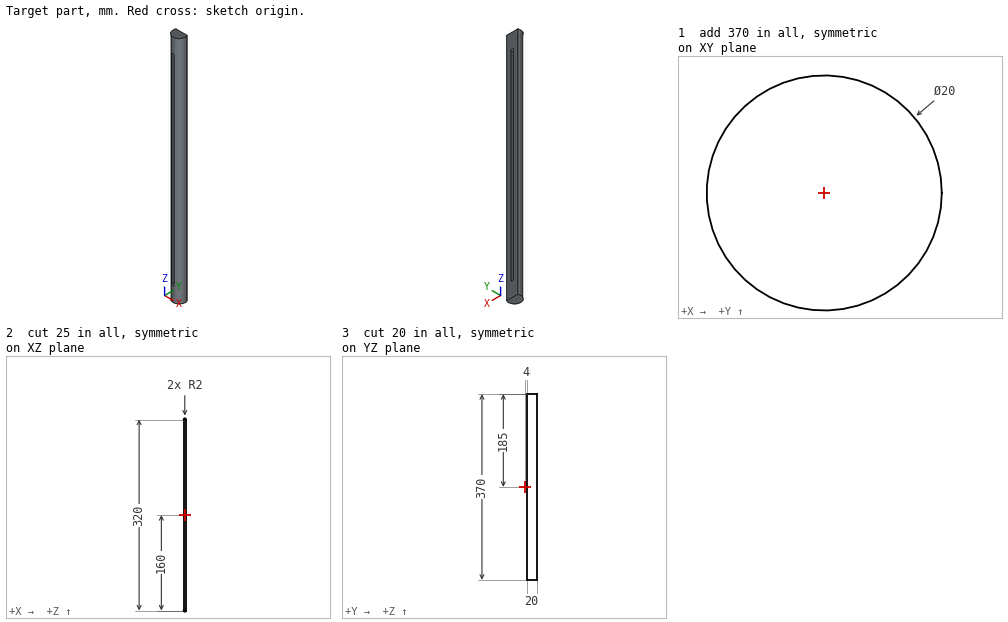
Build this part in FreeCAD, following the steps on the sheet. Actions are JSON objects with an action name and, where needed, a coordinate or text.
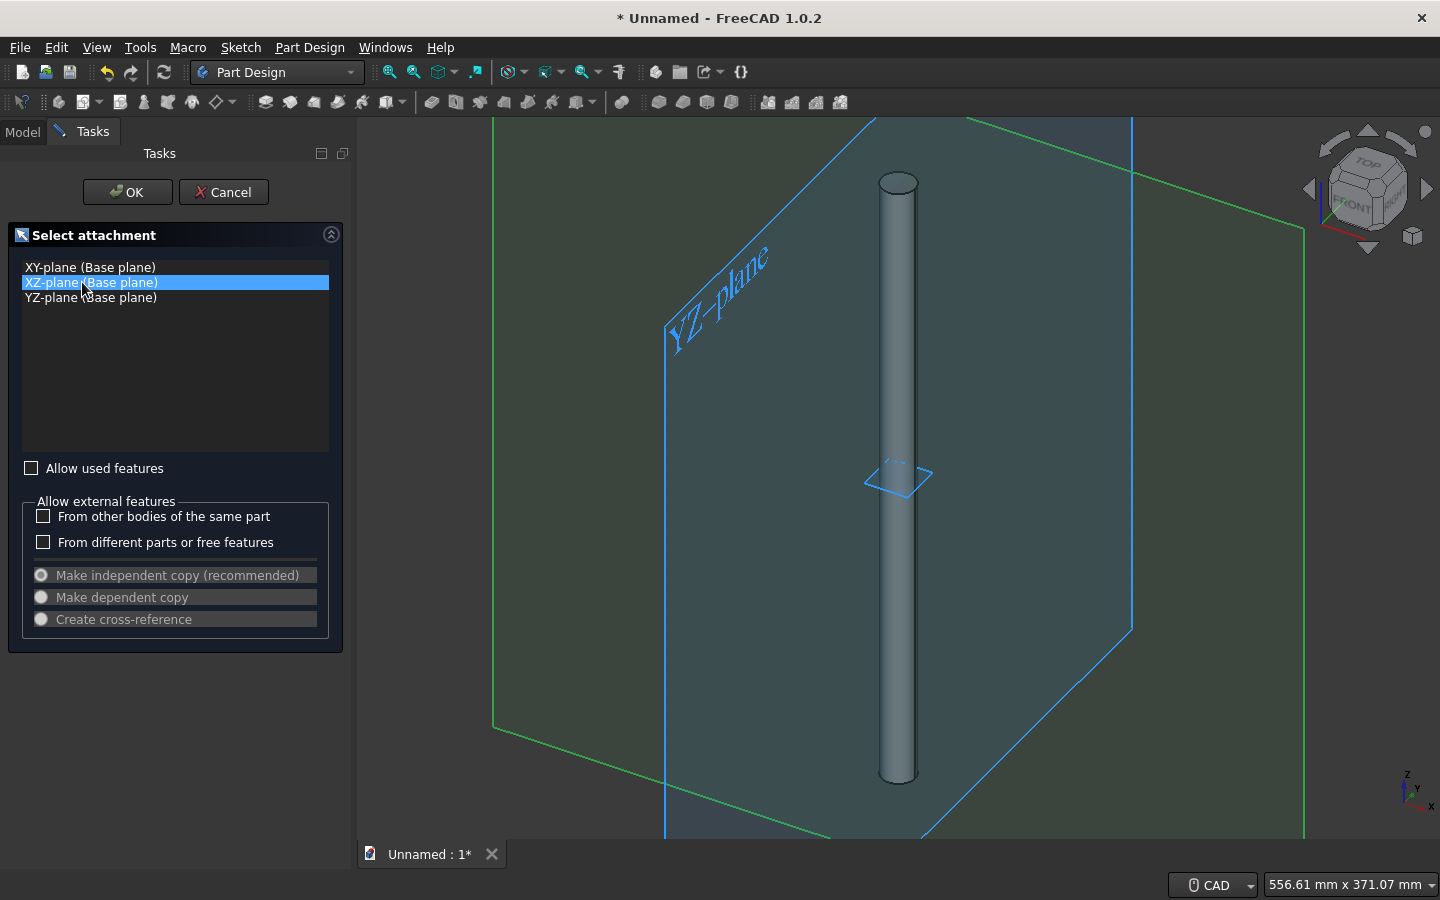
{"action": "left_click", "coordinate": [128, 192]}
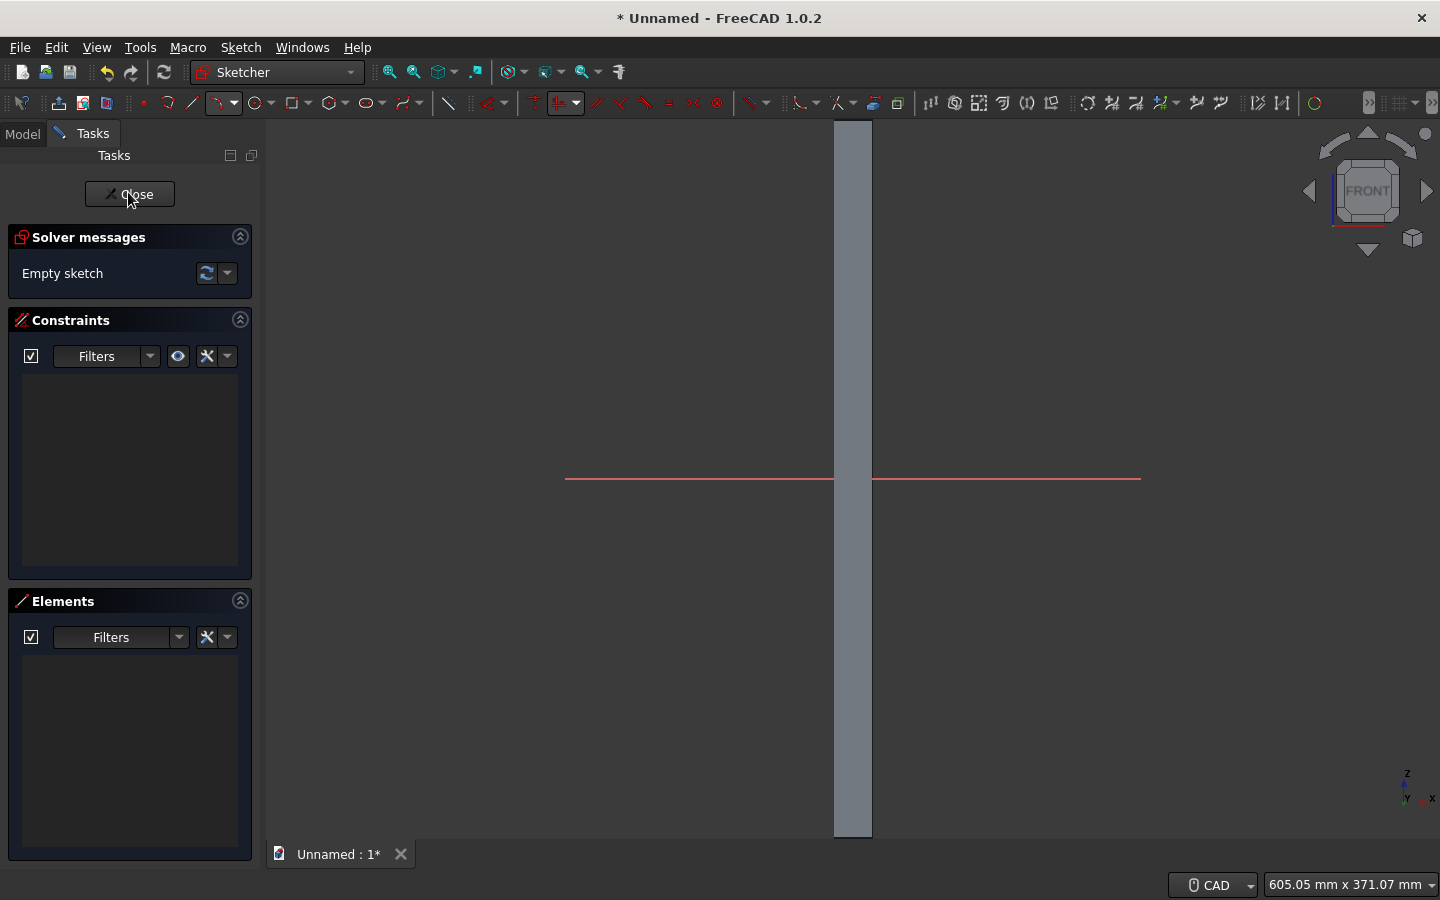
{"action": "left_click", "coordinate": [108, 104]}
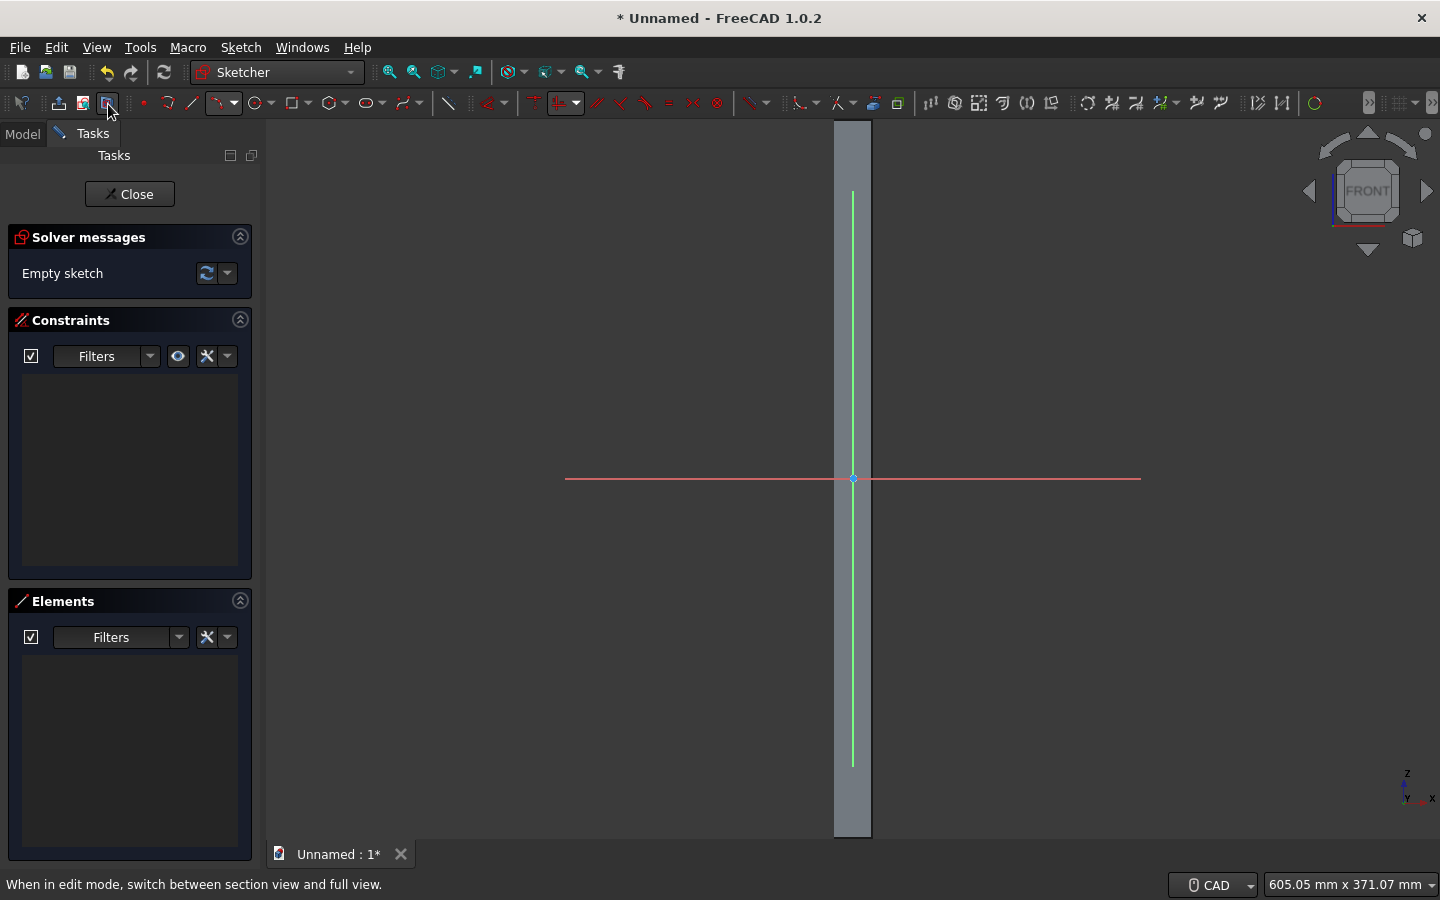
{"action": "scroll", "coordinate": [475, 479], "scroll_direction": "down", "scroll_amount": 1}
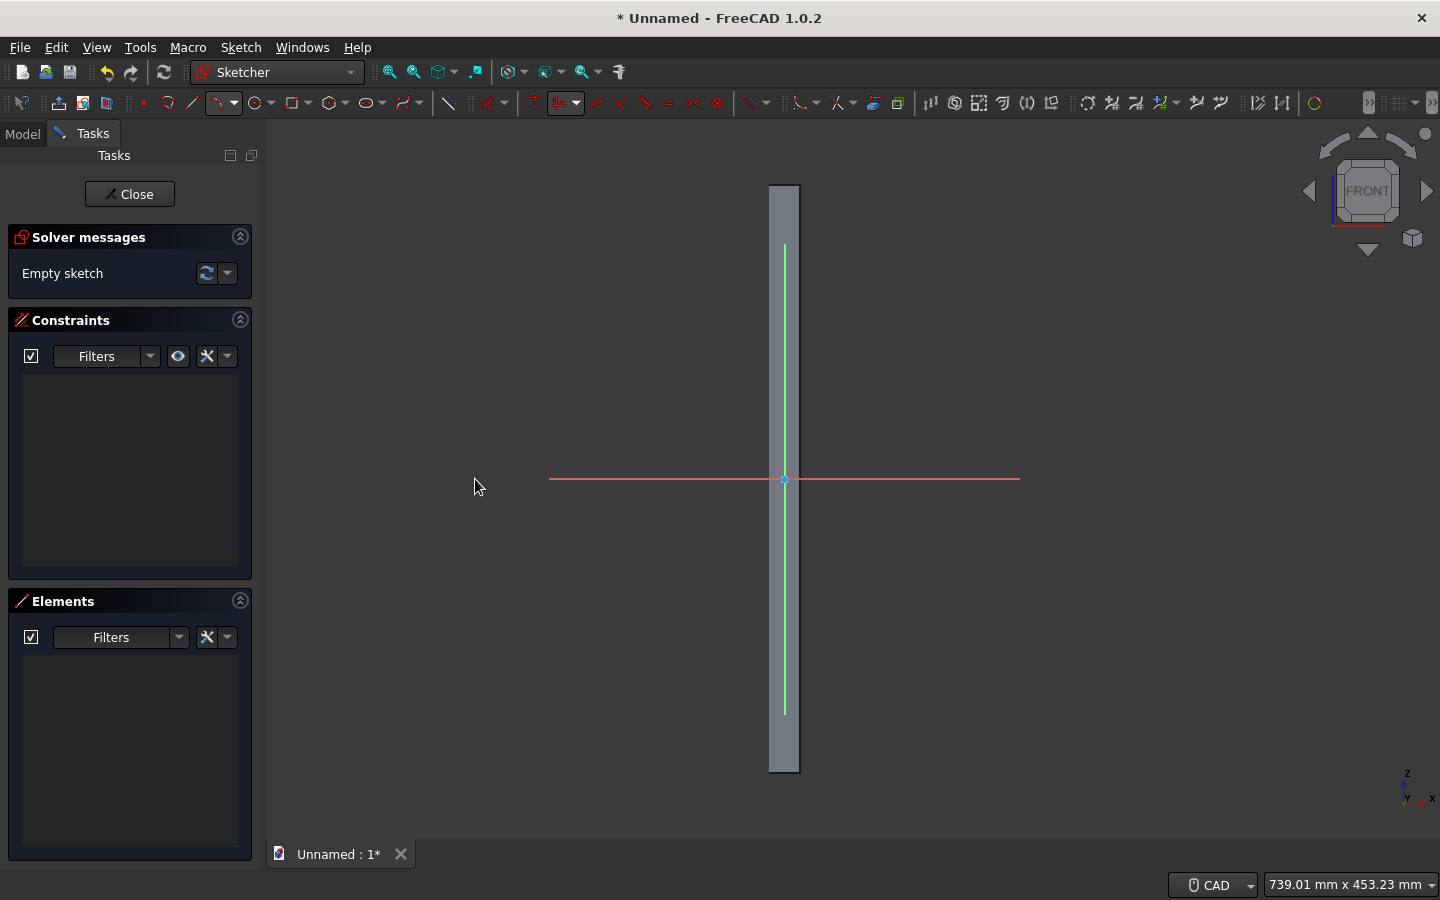
{"action": "left_click", "coordinate": [366, 104]}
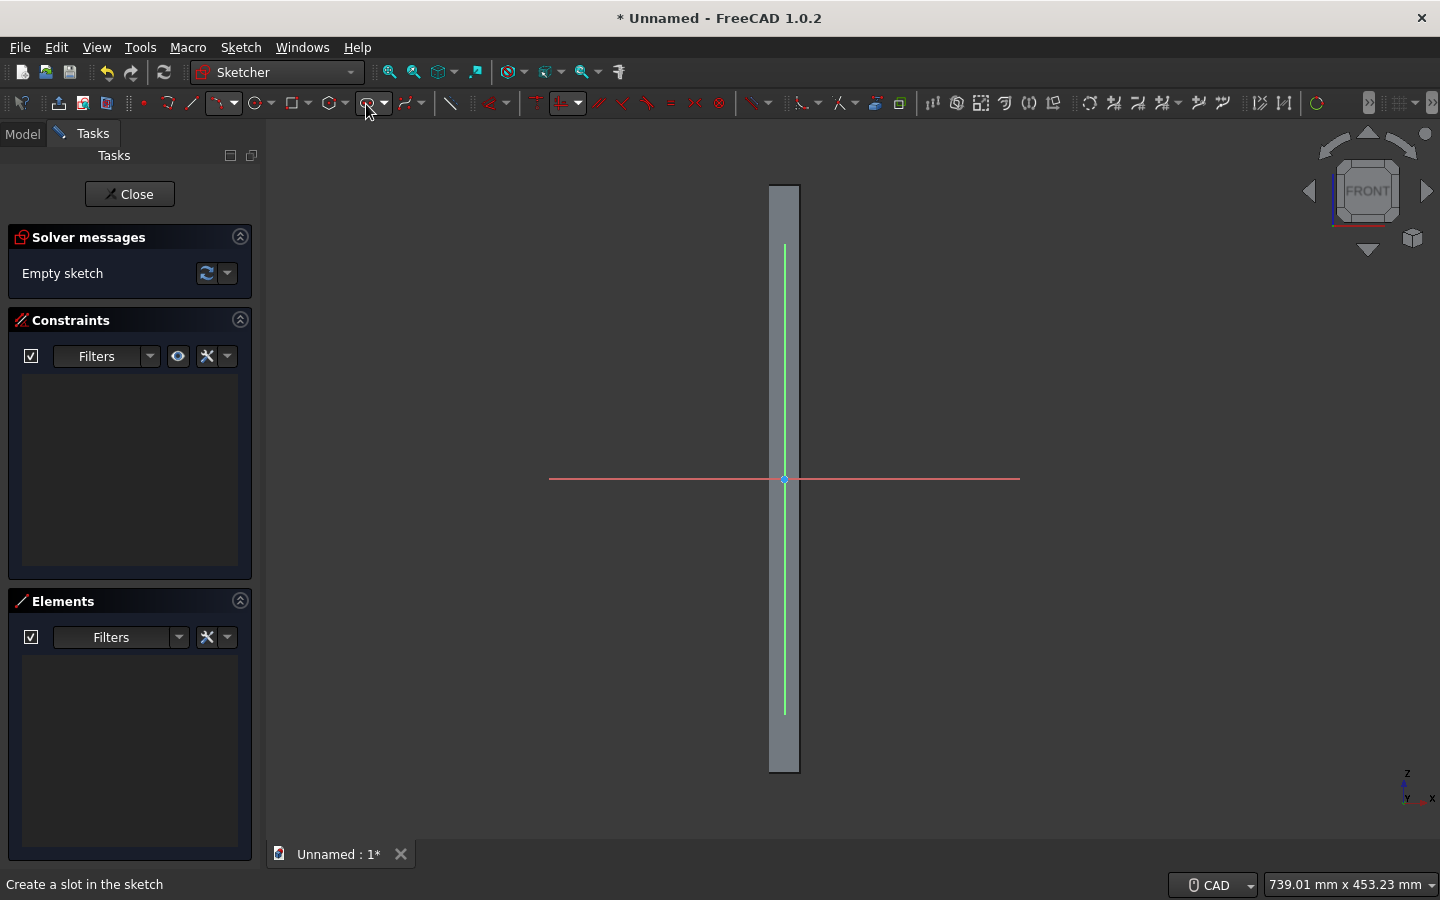
{"action": "scroll", "coordinate": [785, 733], "scroll_direction": "up", "scroll_amount": 10}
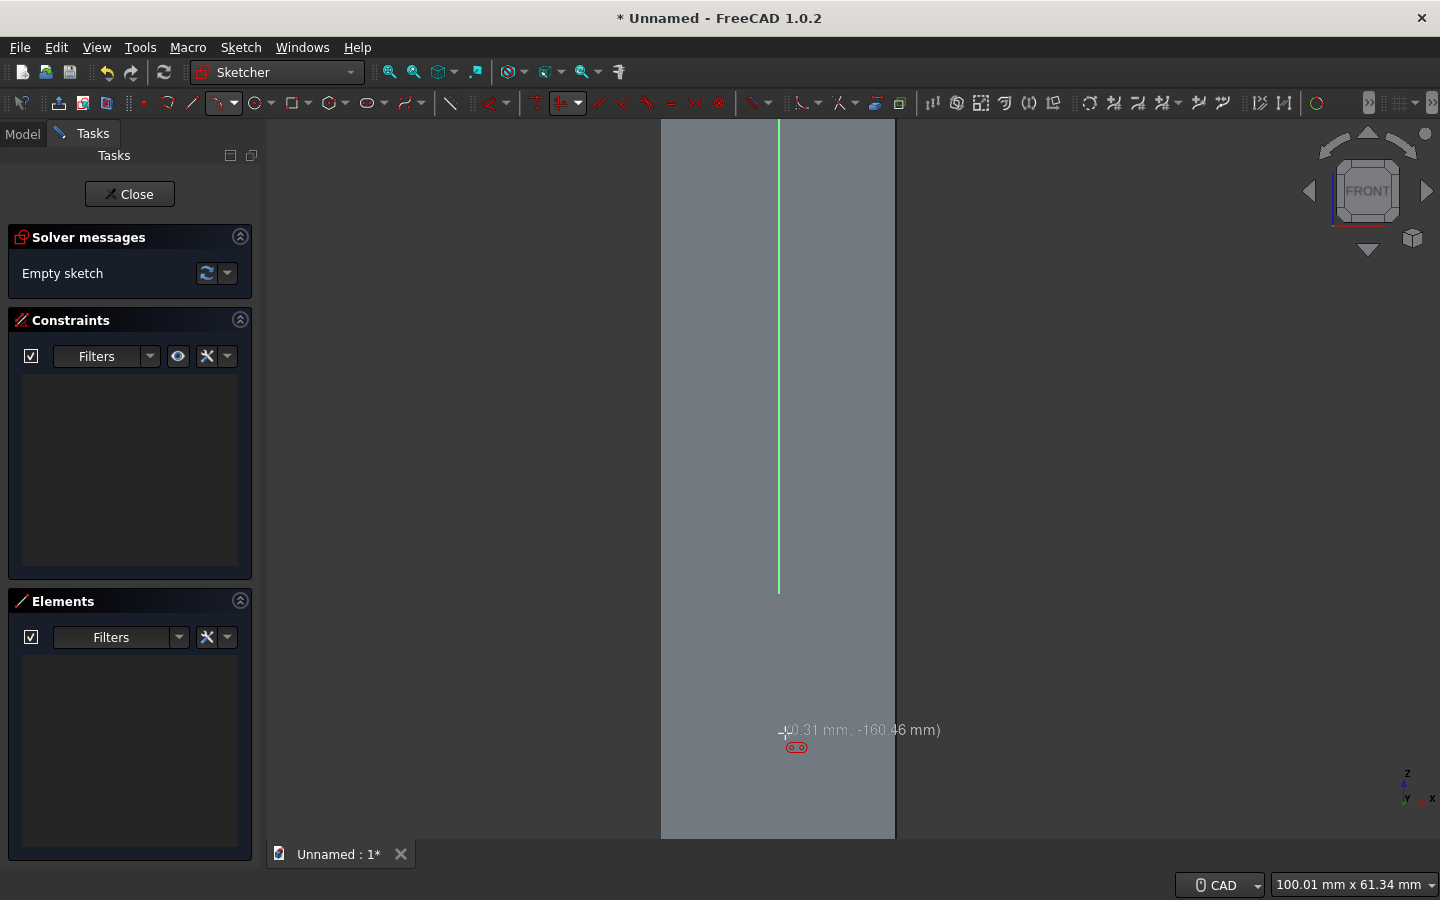
{"action": "scroll", "coordinate": [785, 734], "scroll_direction": "down", "scroll_amount": 10}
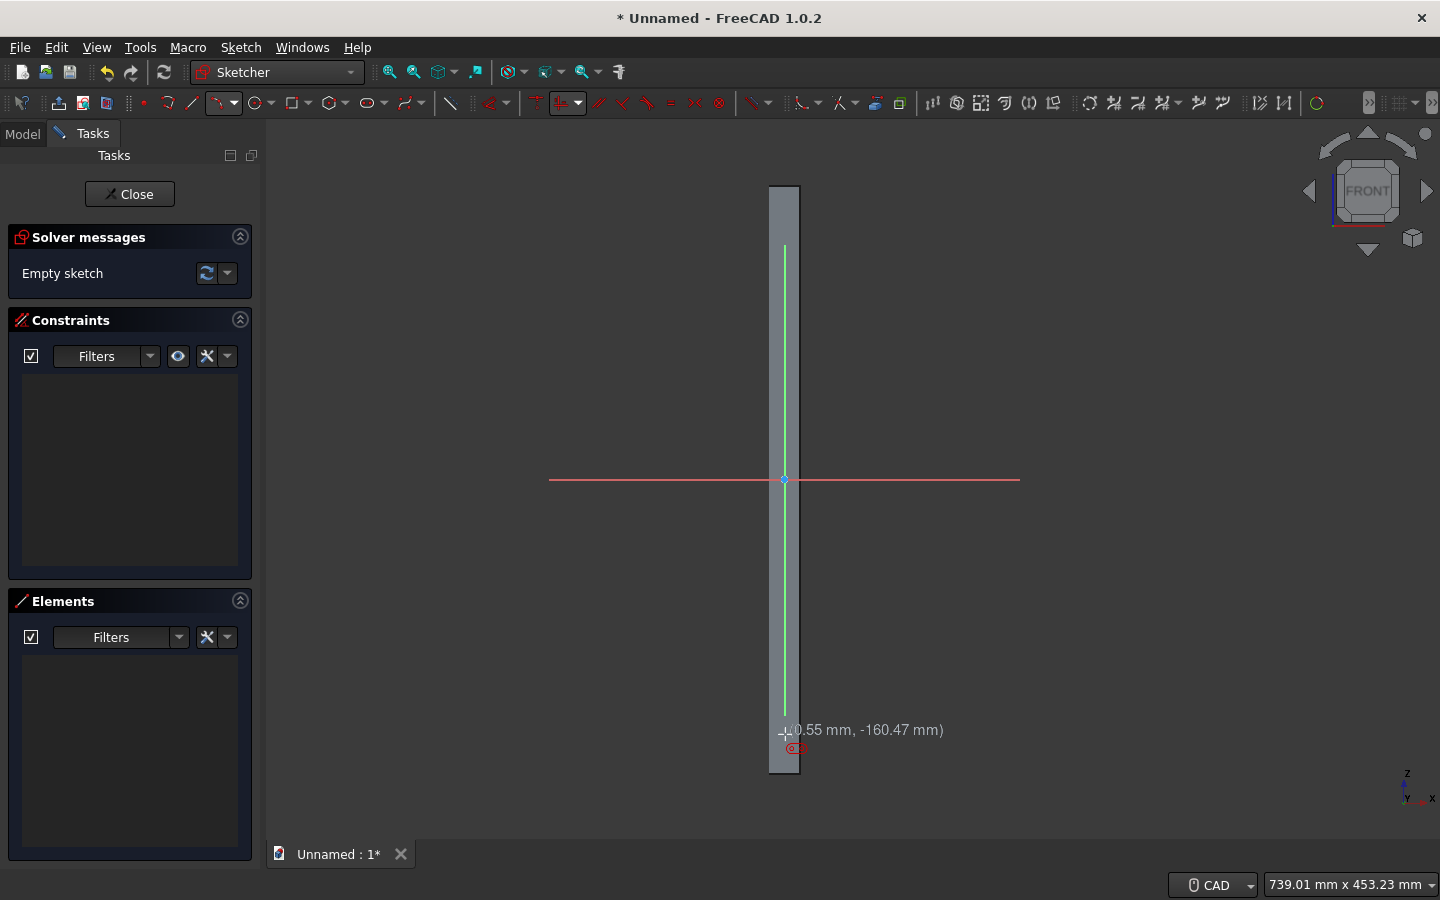
{"action": "left_click", "coordinate": [785, 734]}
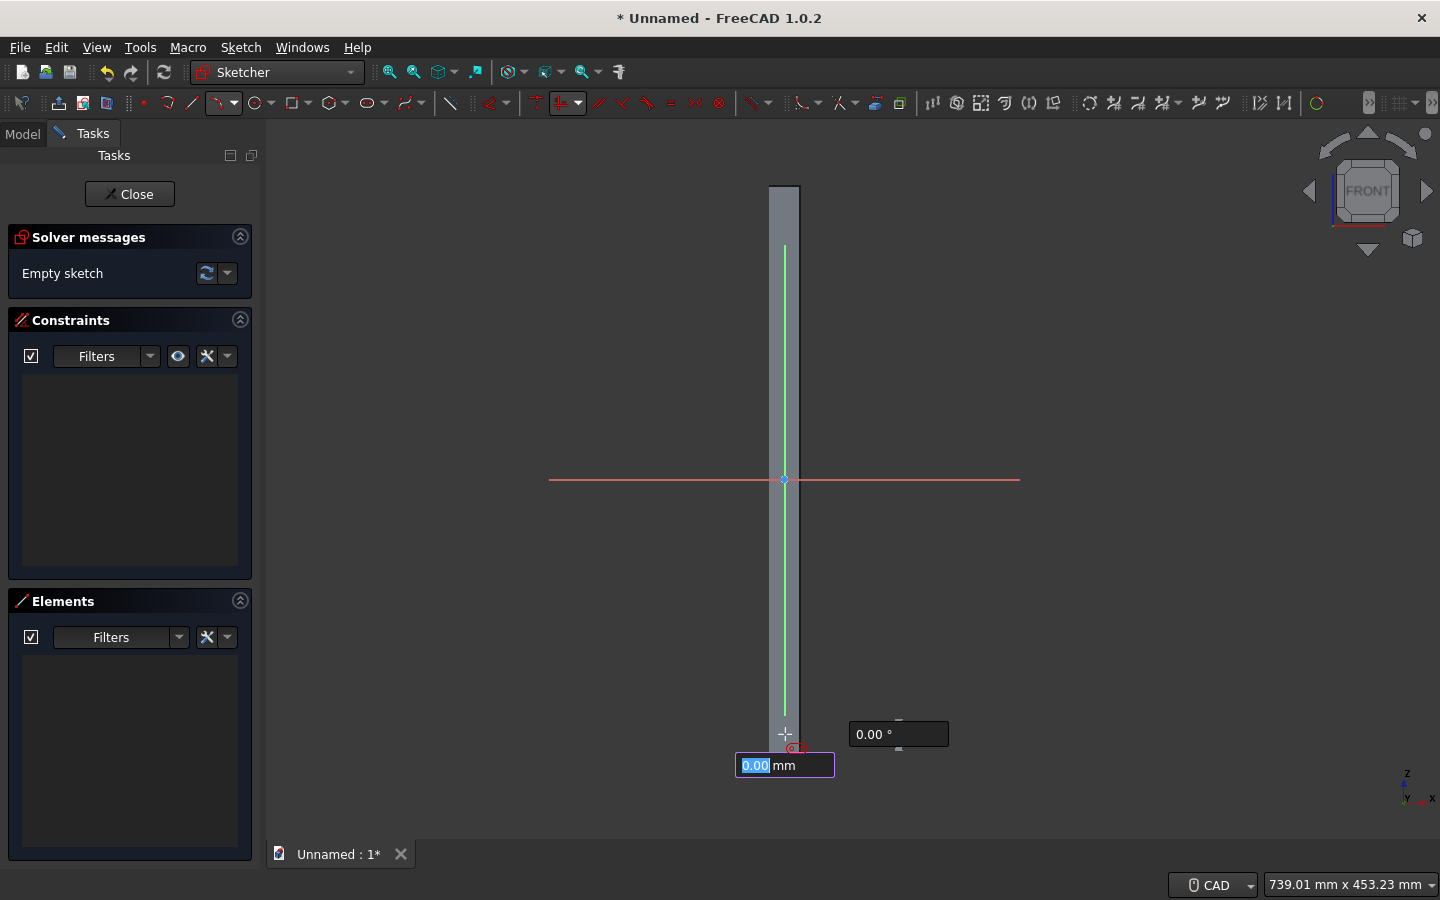
{"action": "left_click", "coordinate": [794, 226]}